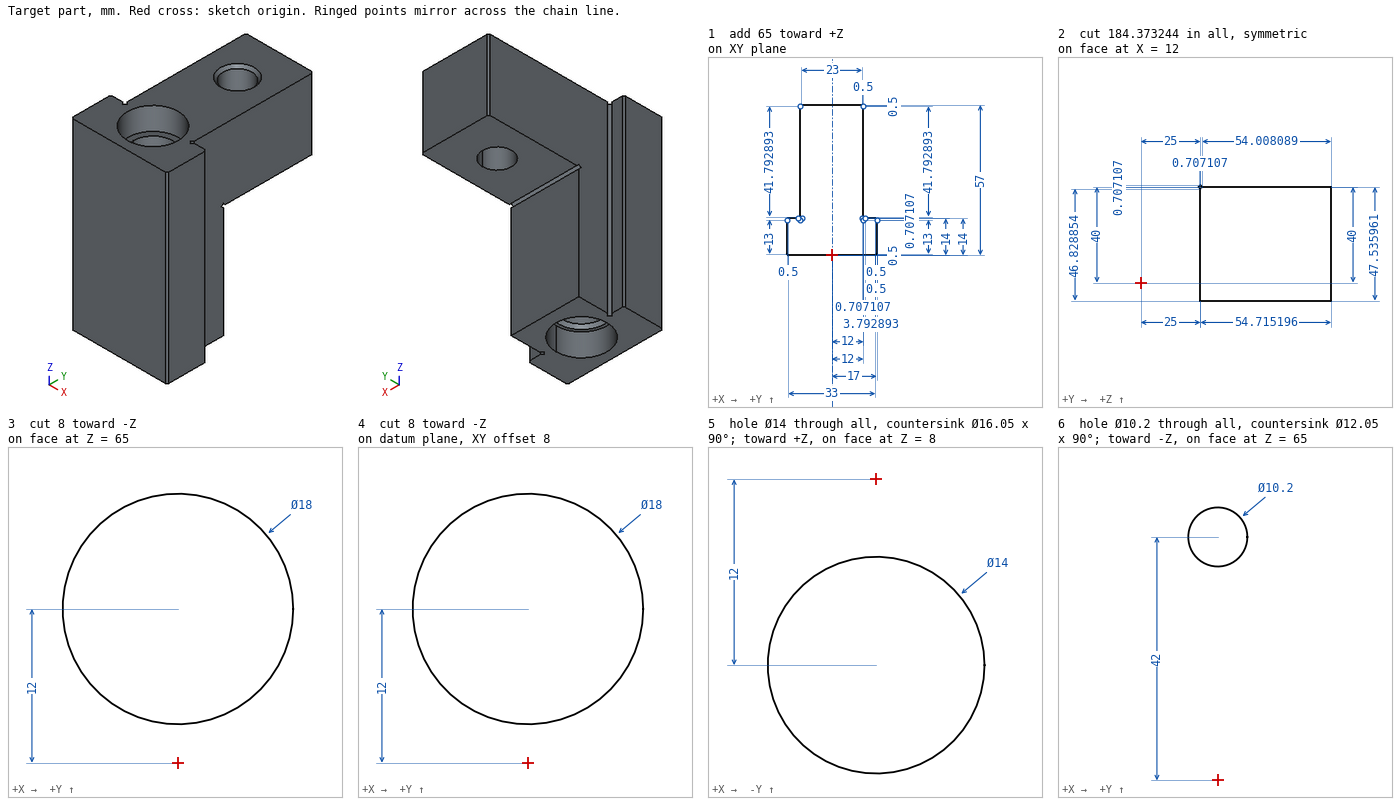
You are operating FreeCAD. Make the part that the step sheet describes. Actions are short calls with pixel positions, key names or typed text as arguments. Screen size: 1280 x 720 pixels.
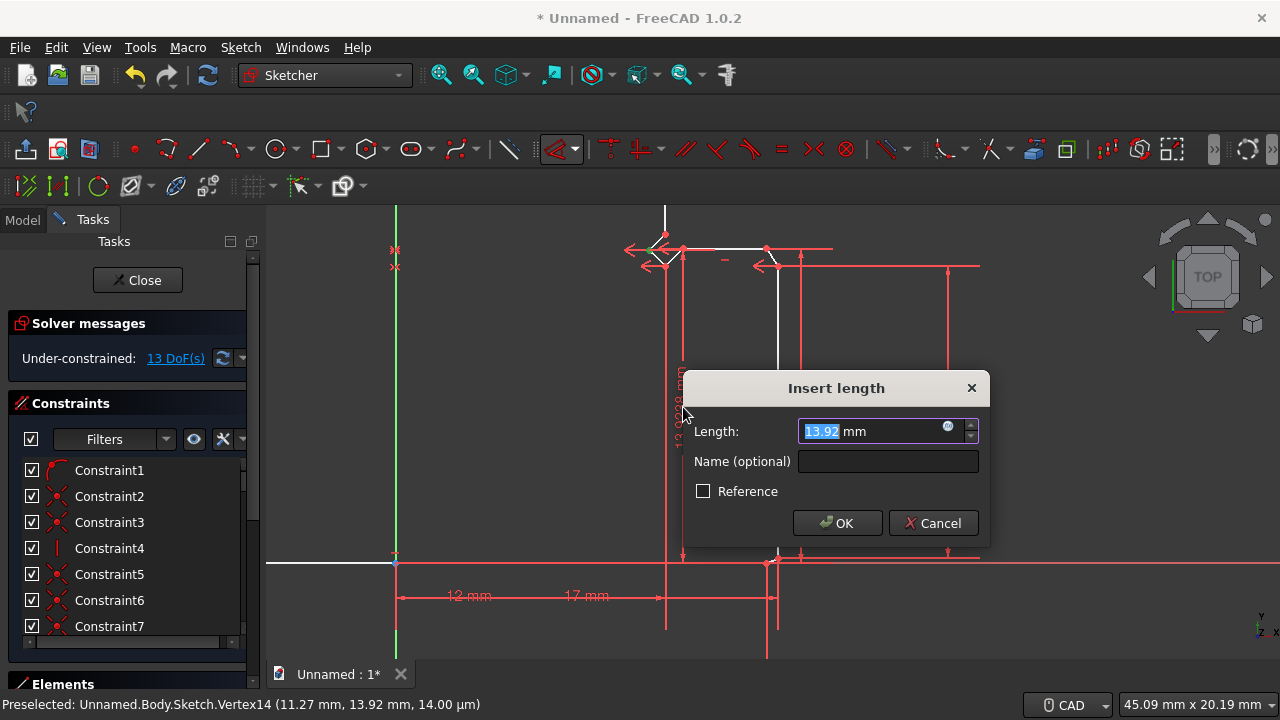
text(14)
key(Return)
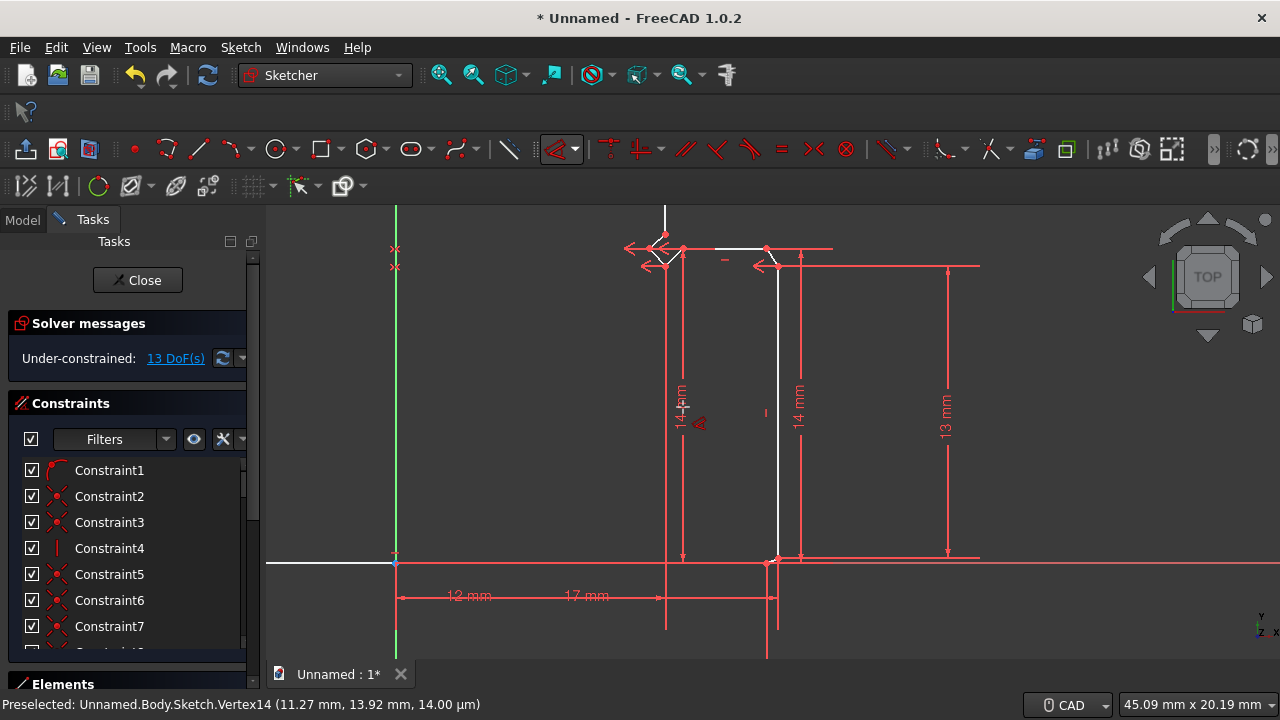
click(665, 234)
click(531, 621)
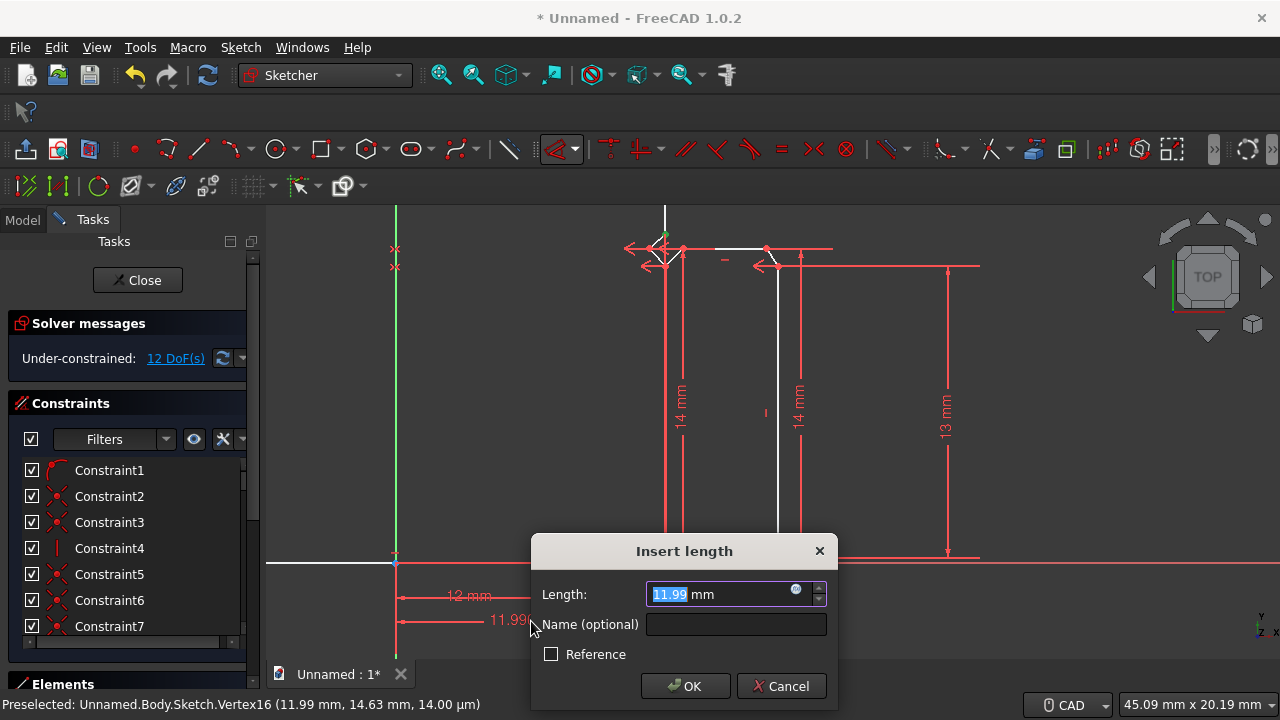
text(12)
key(Return)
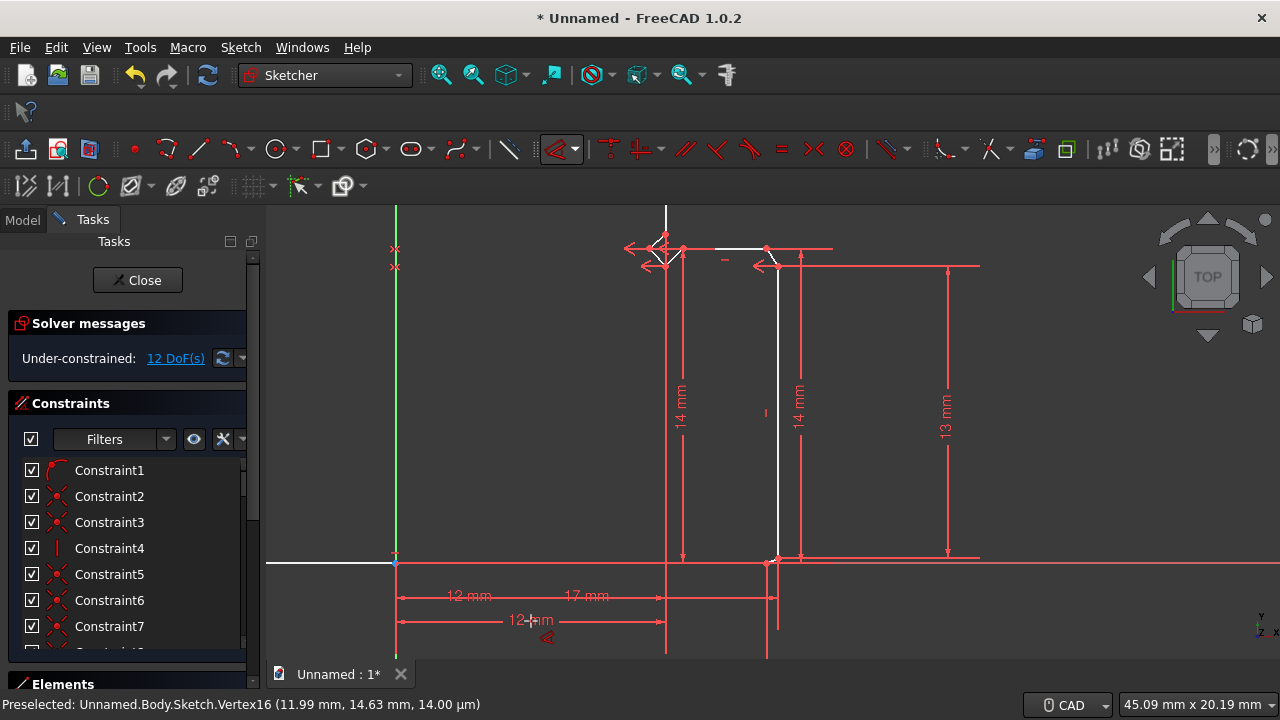
scroll(783, 561, down, 8)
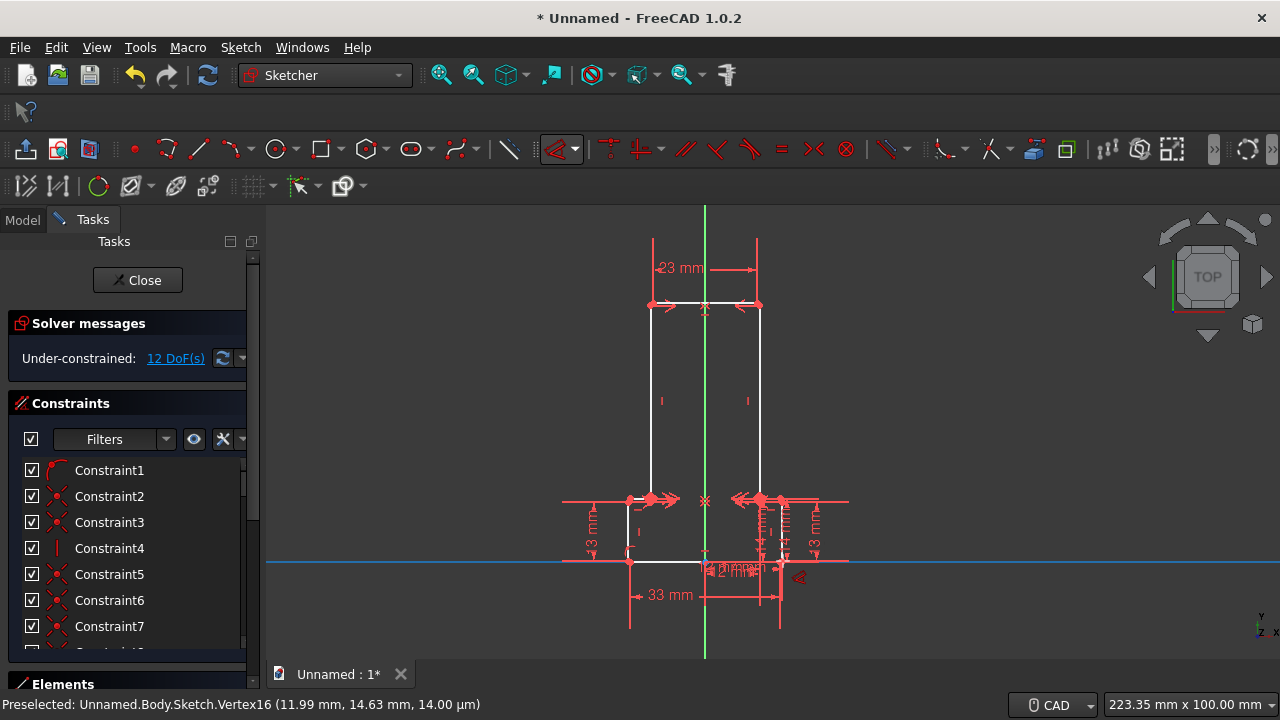
scroll(757, 303, up, 7)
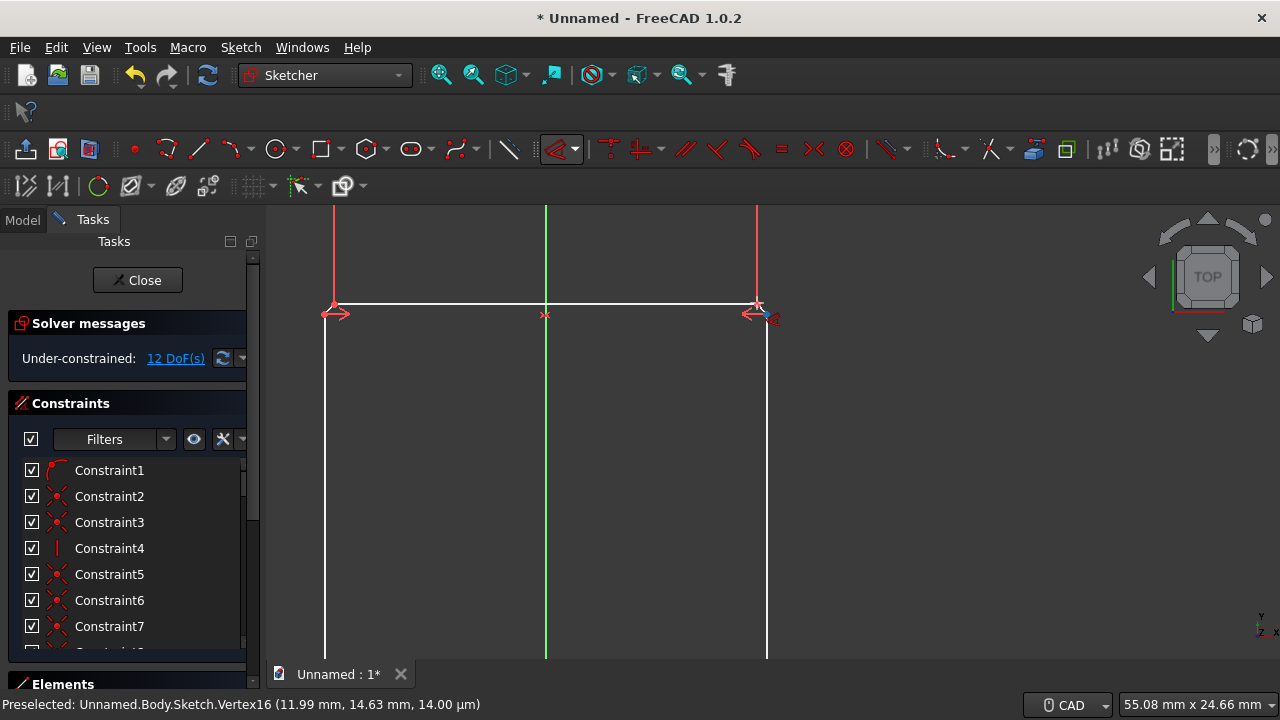
click(757, 304)
click(791, 468)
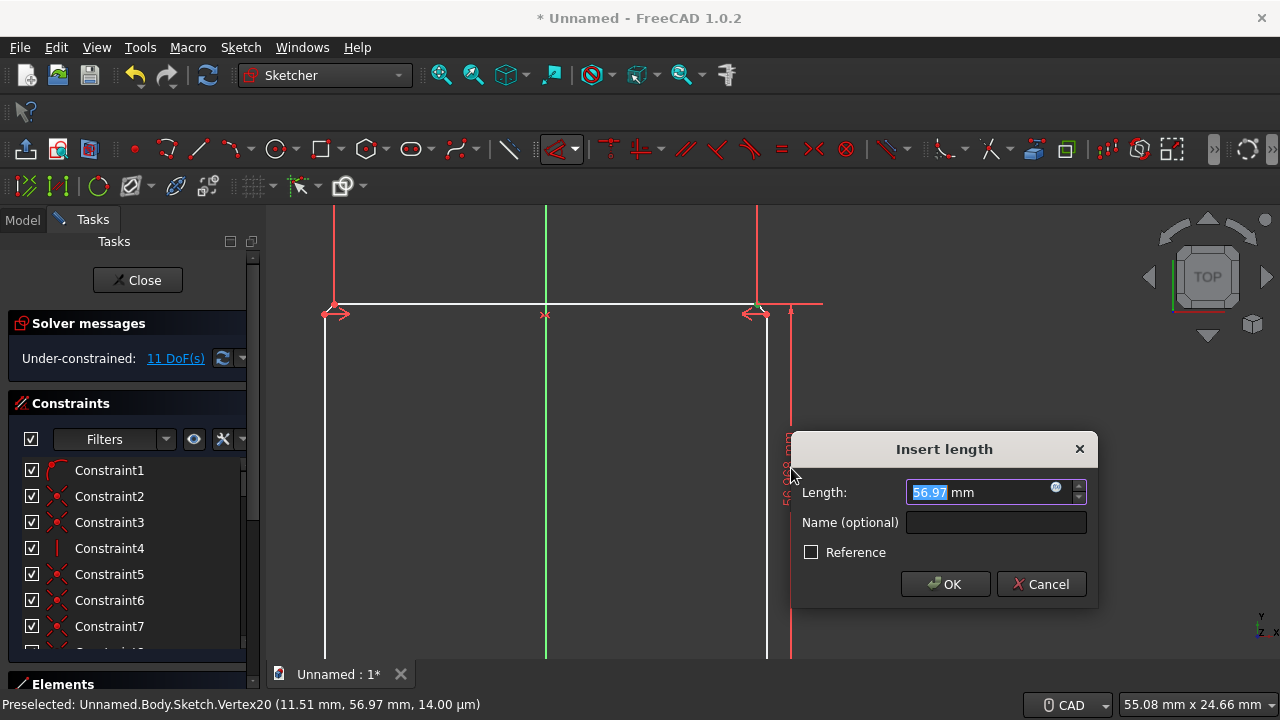
text(57)
key(Return)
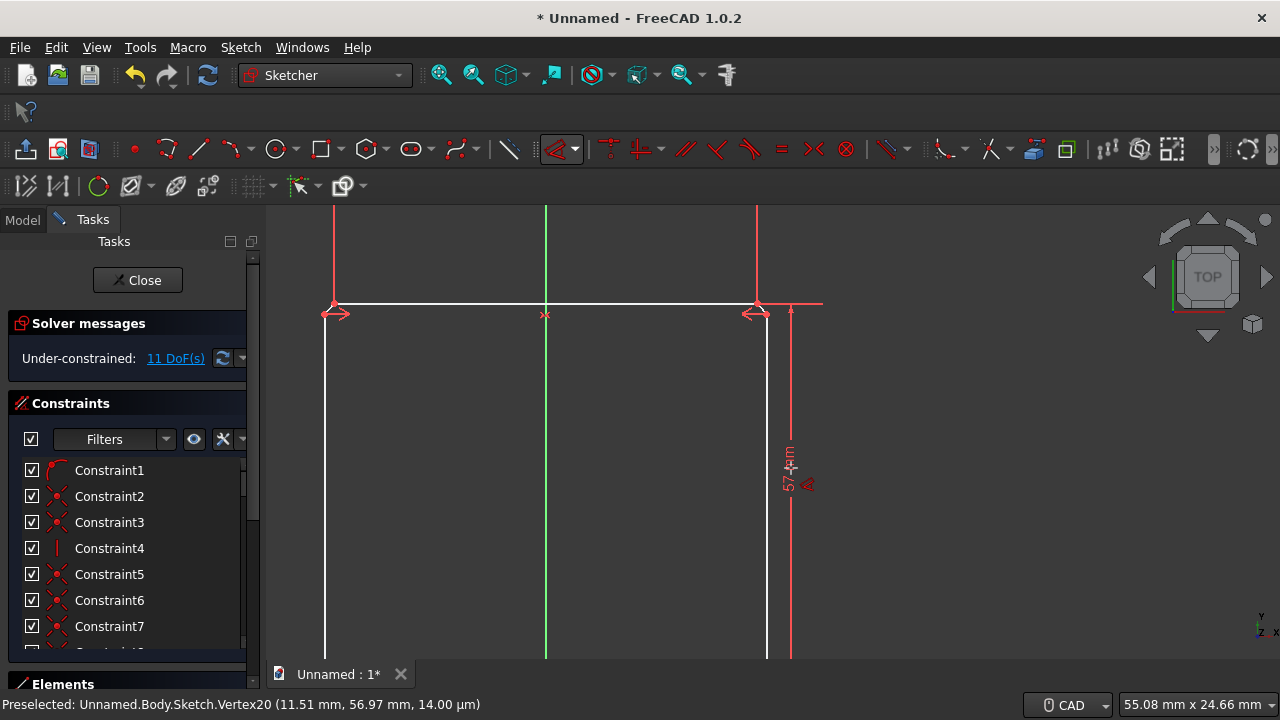
scroll(756, 302, down, 7)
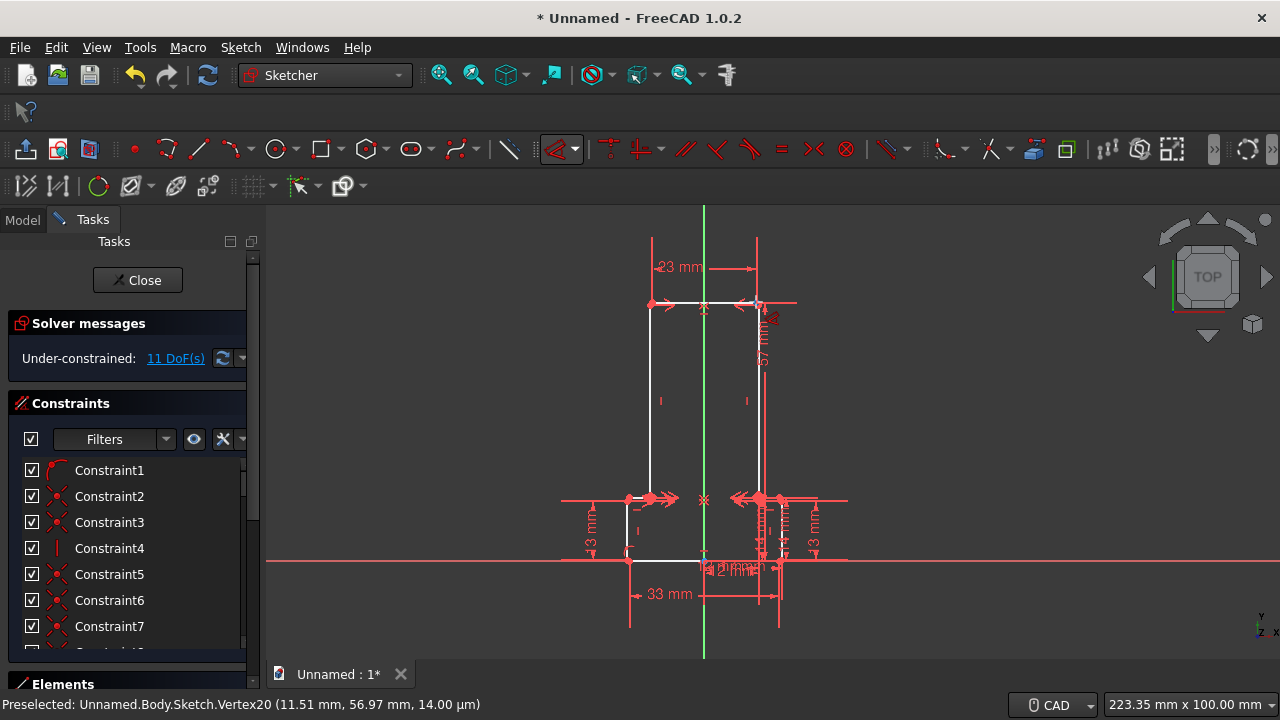
scroll(782, 560, up, 15)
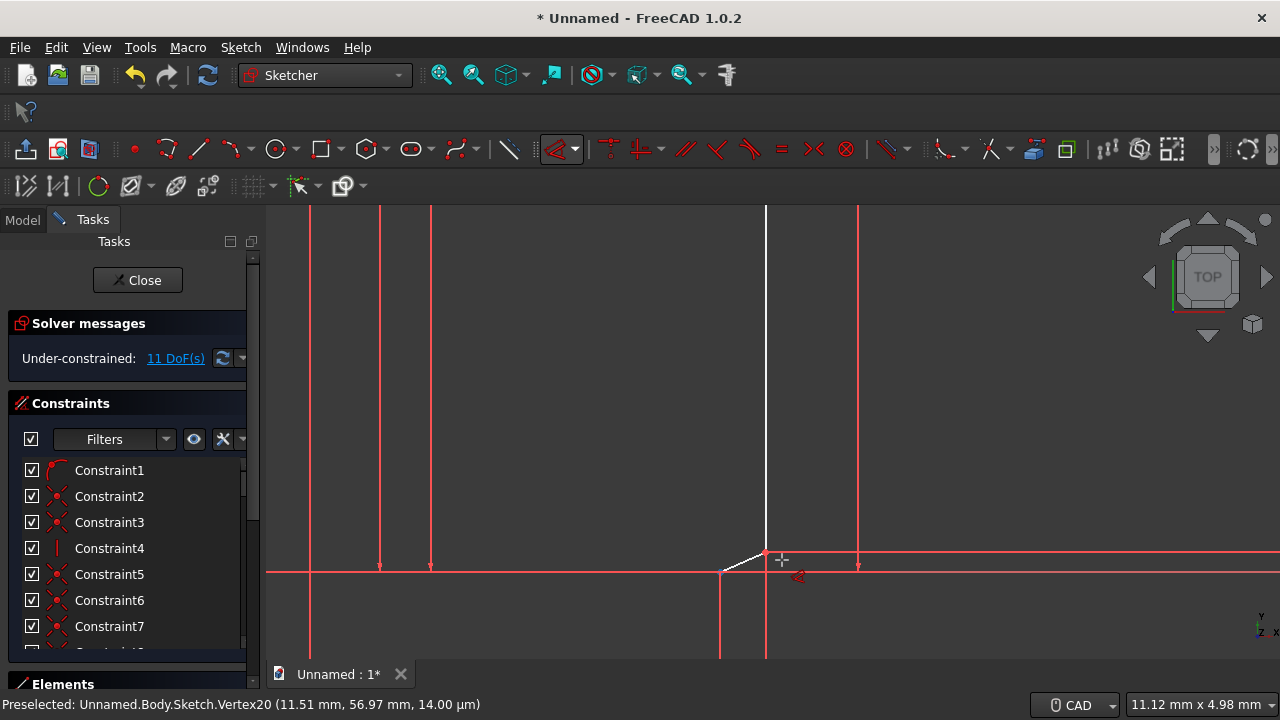
click(766, 552)
click(800, 558)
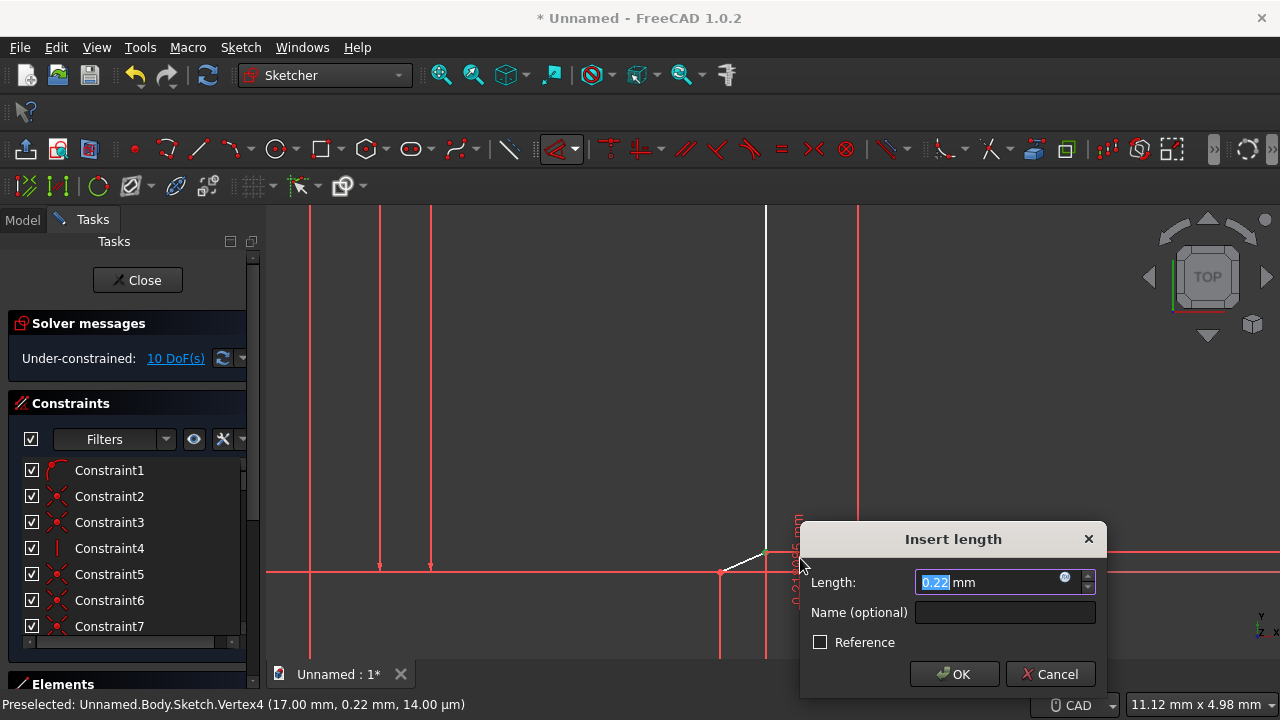
text(0.5)
key(Return)